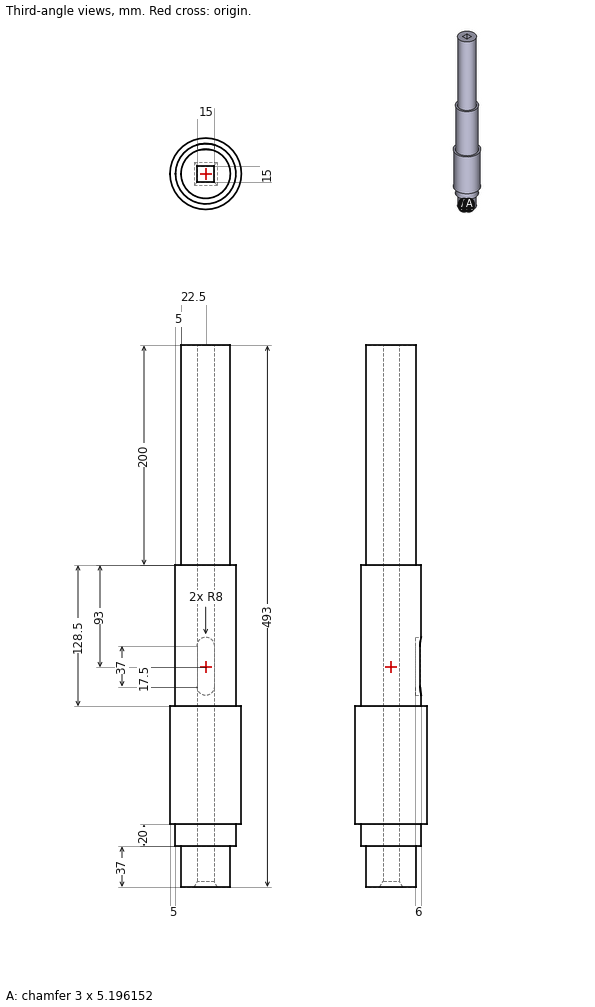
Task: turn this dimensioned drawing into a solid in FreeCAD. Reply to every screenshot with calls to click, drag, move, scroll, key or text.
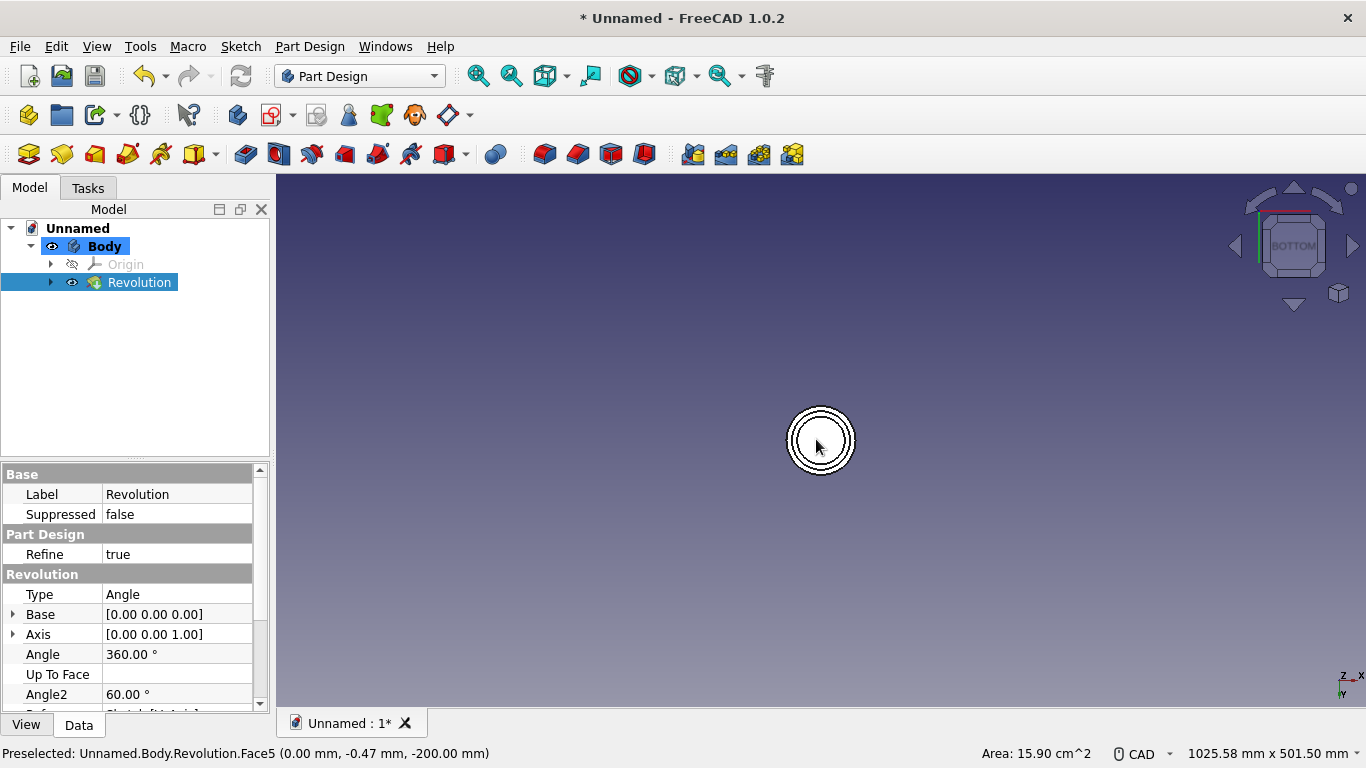
click(270, 116)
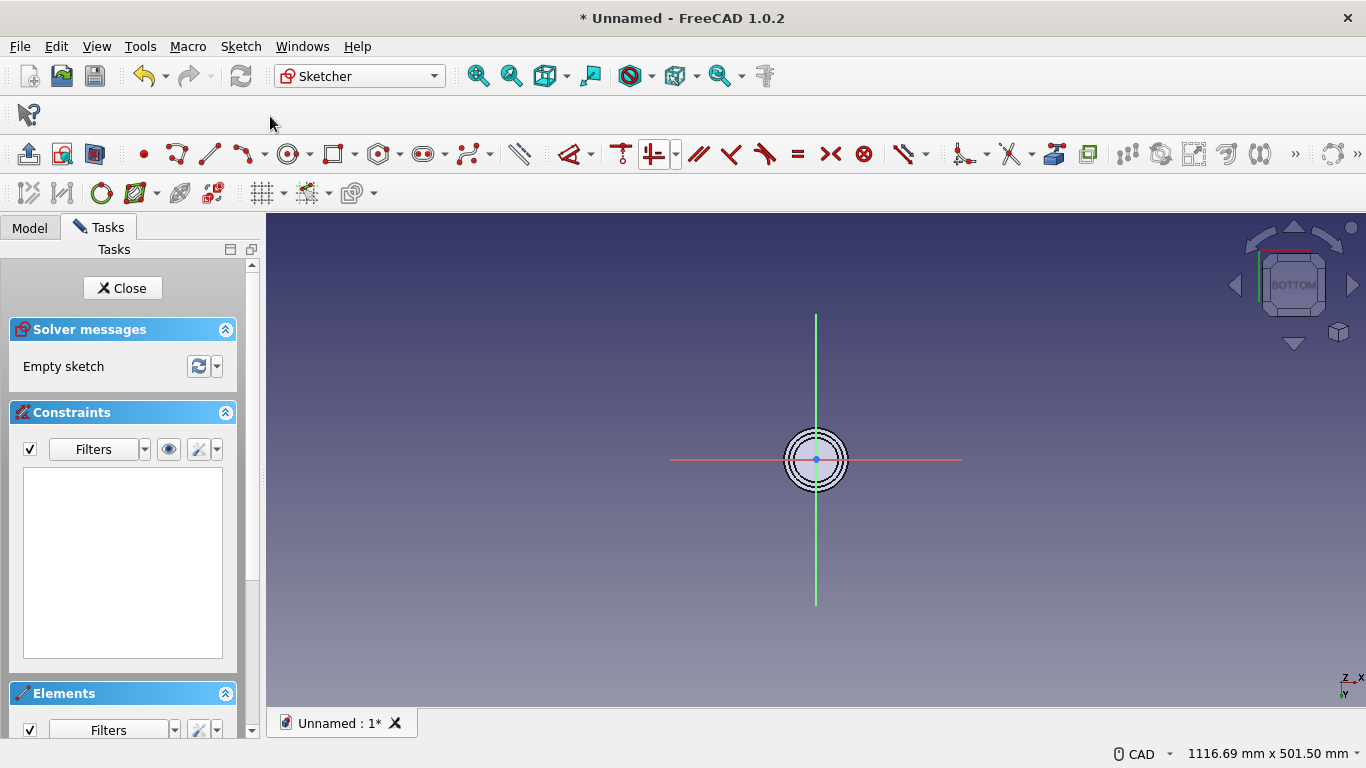
scroll(820, 460, up, 15)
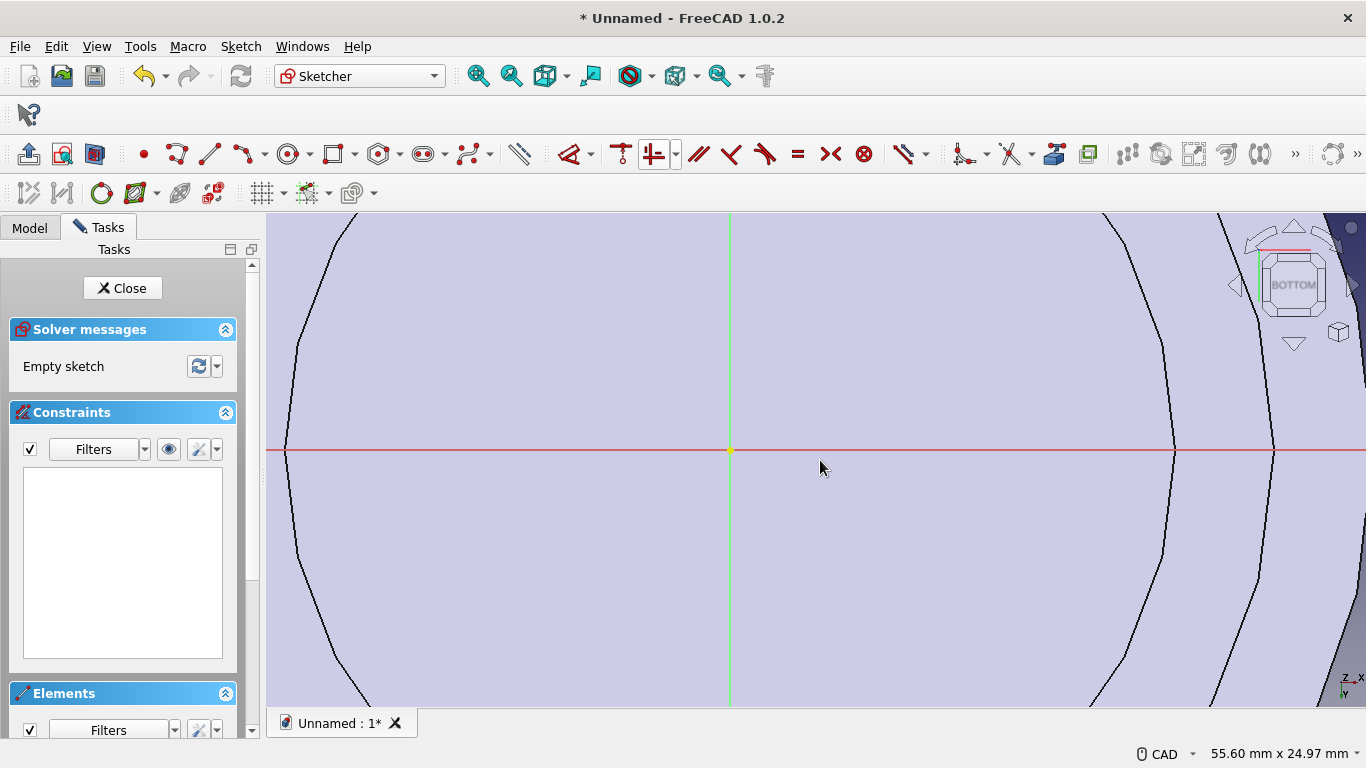
key(g)
key(v)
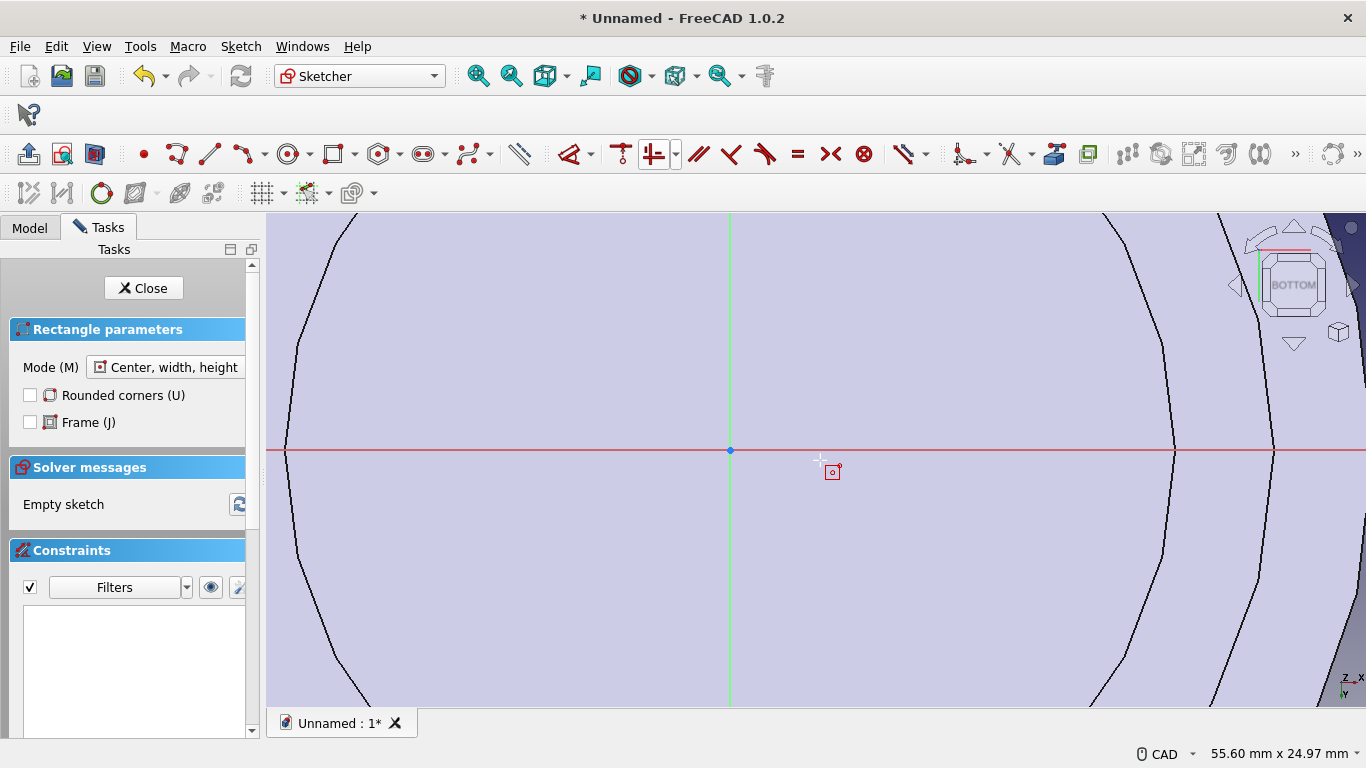
click(730, 450)
move(878, 302)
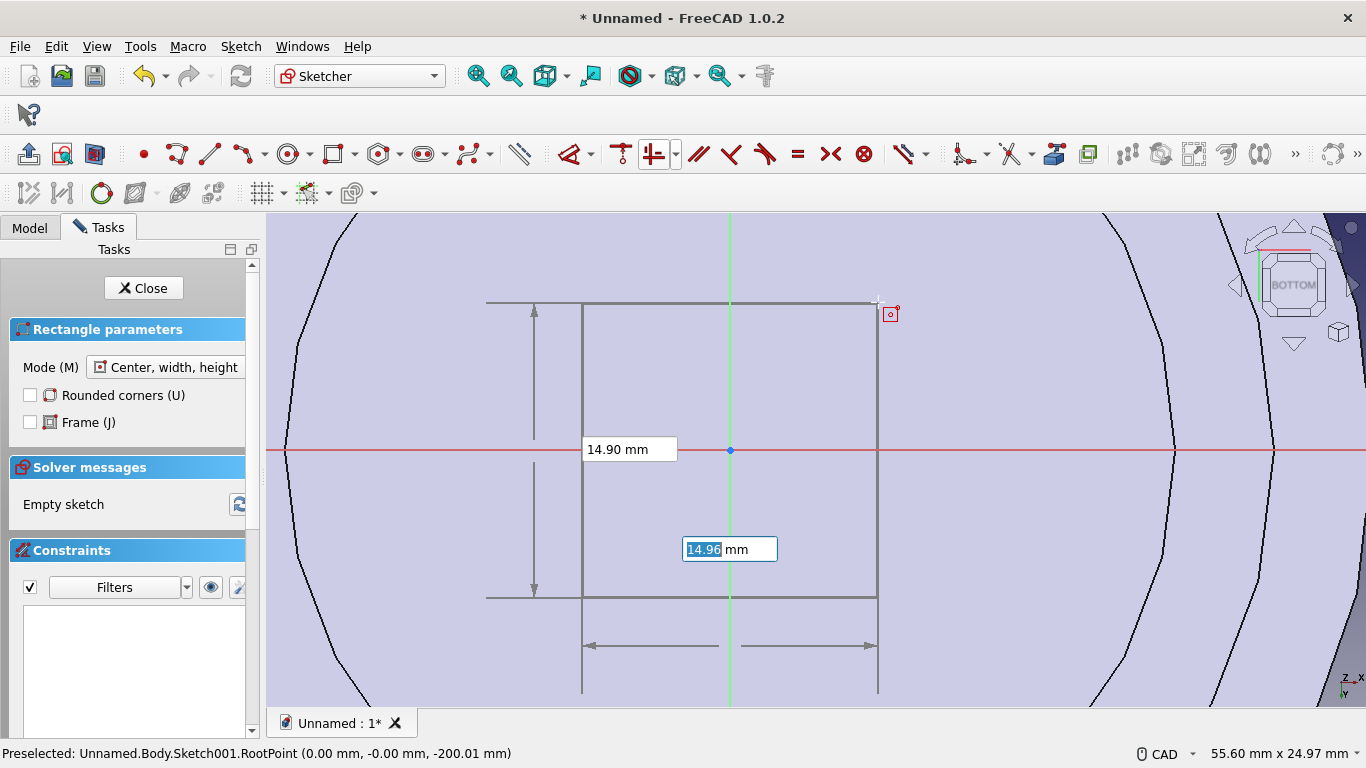
text(15)
key(Tab)
text(15)
key(Return)
key(Escape)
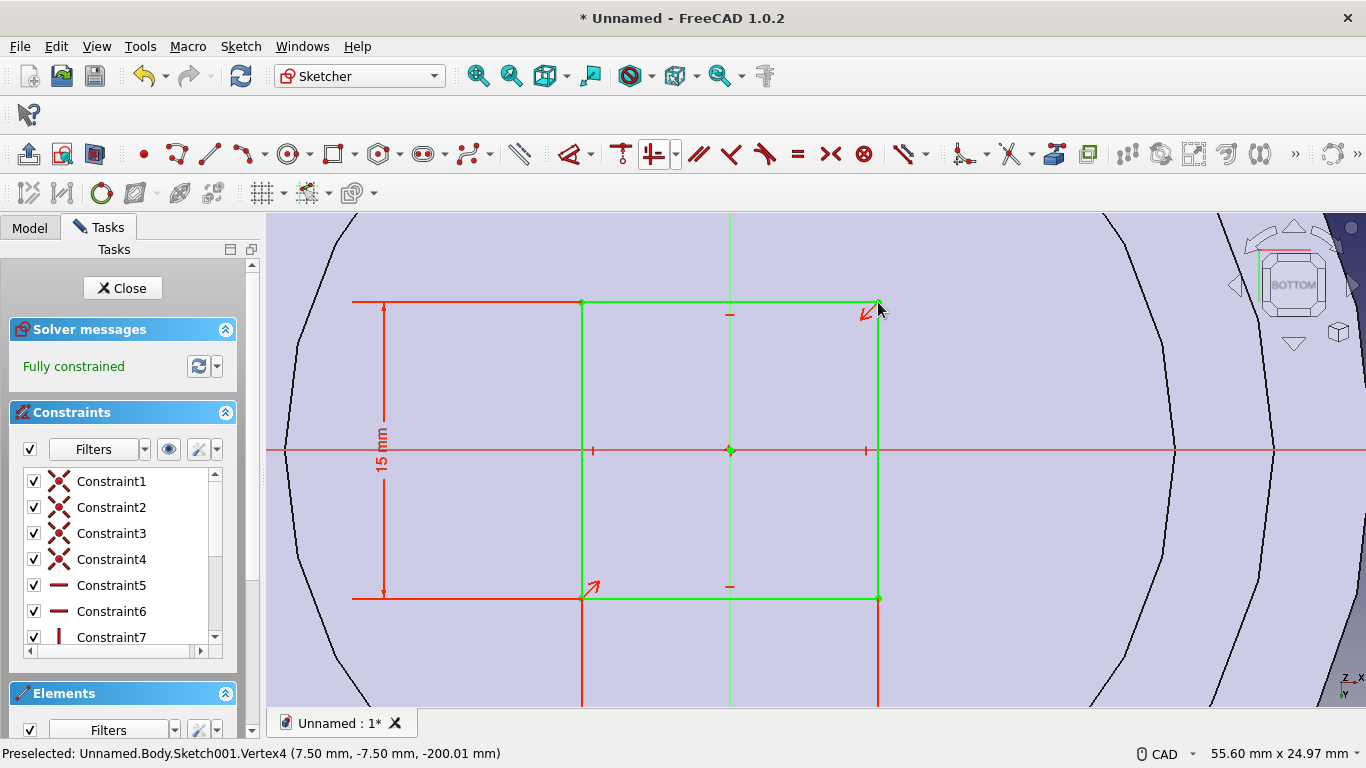
click(123, 288)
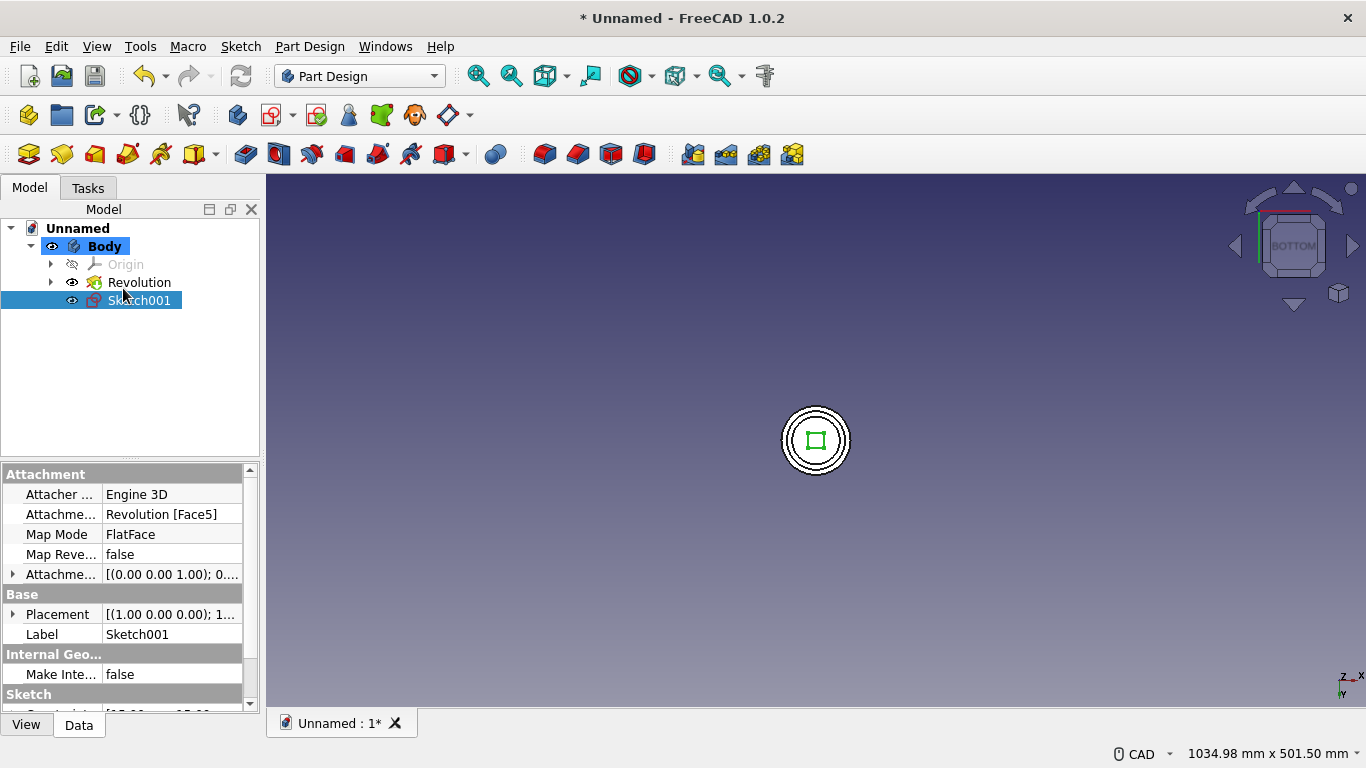
click(246, 154)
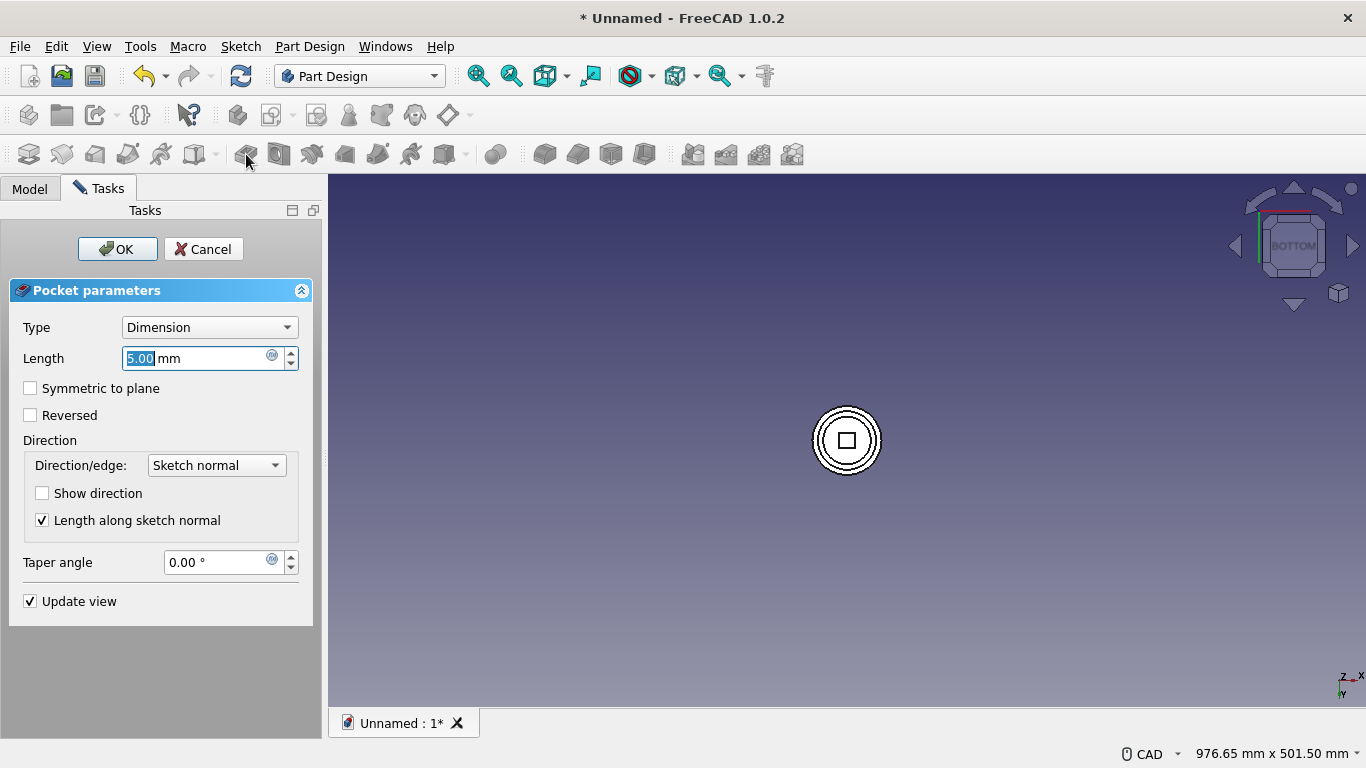
click(210, 328)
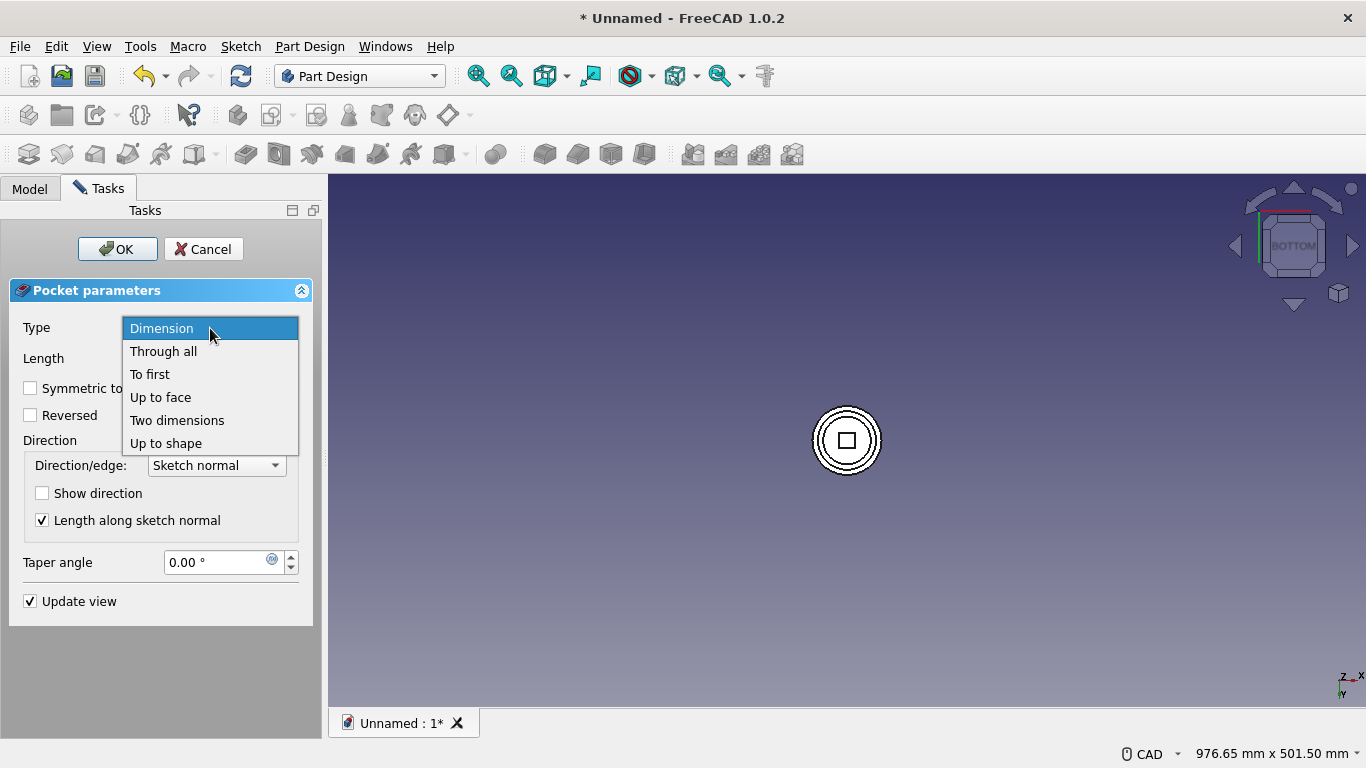
click(208, 352)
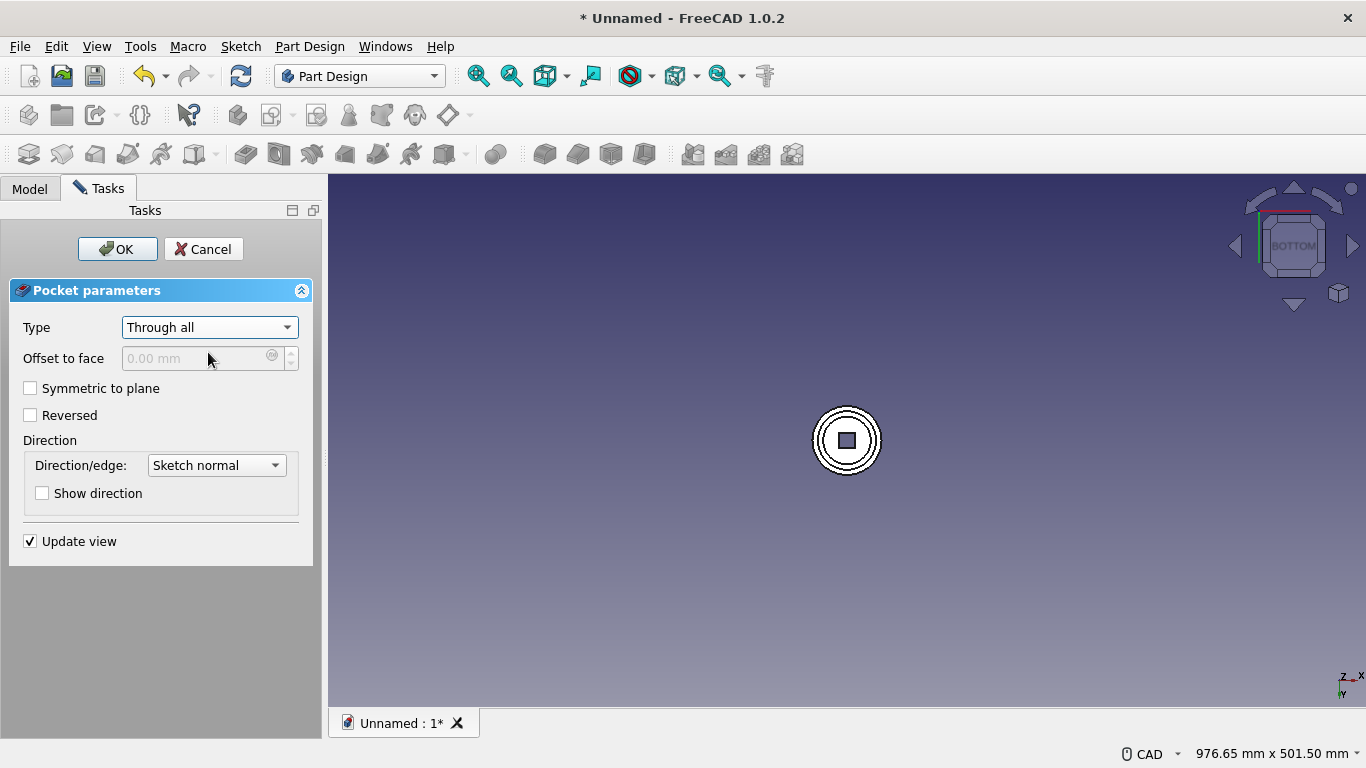
click(118, 249)